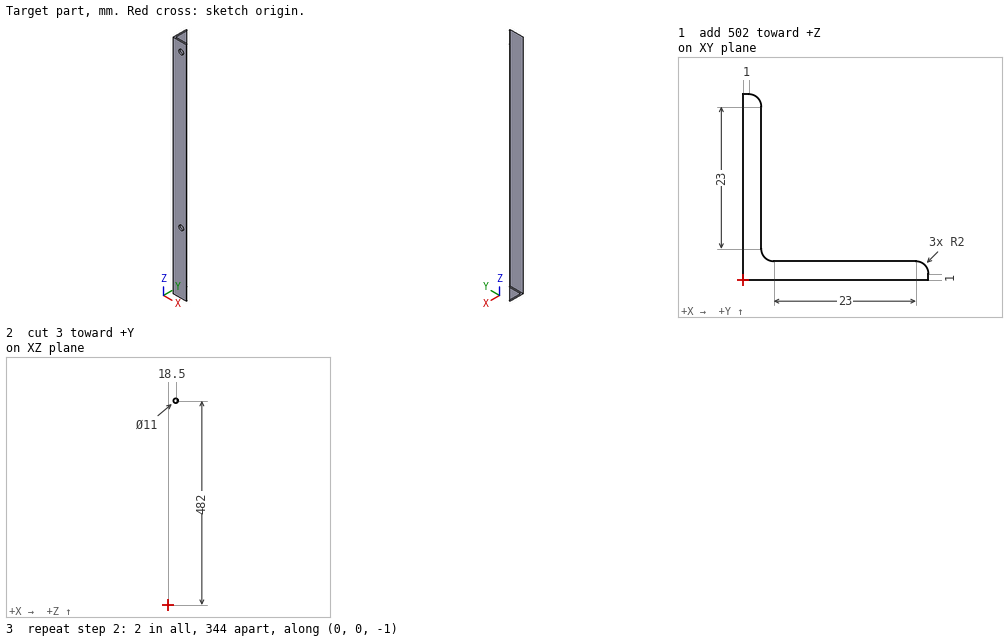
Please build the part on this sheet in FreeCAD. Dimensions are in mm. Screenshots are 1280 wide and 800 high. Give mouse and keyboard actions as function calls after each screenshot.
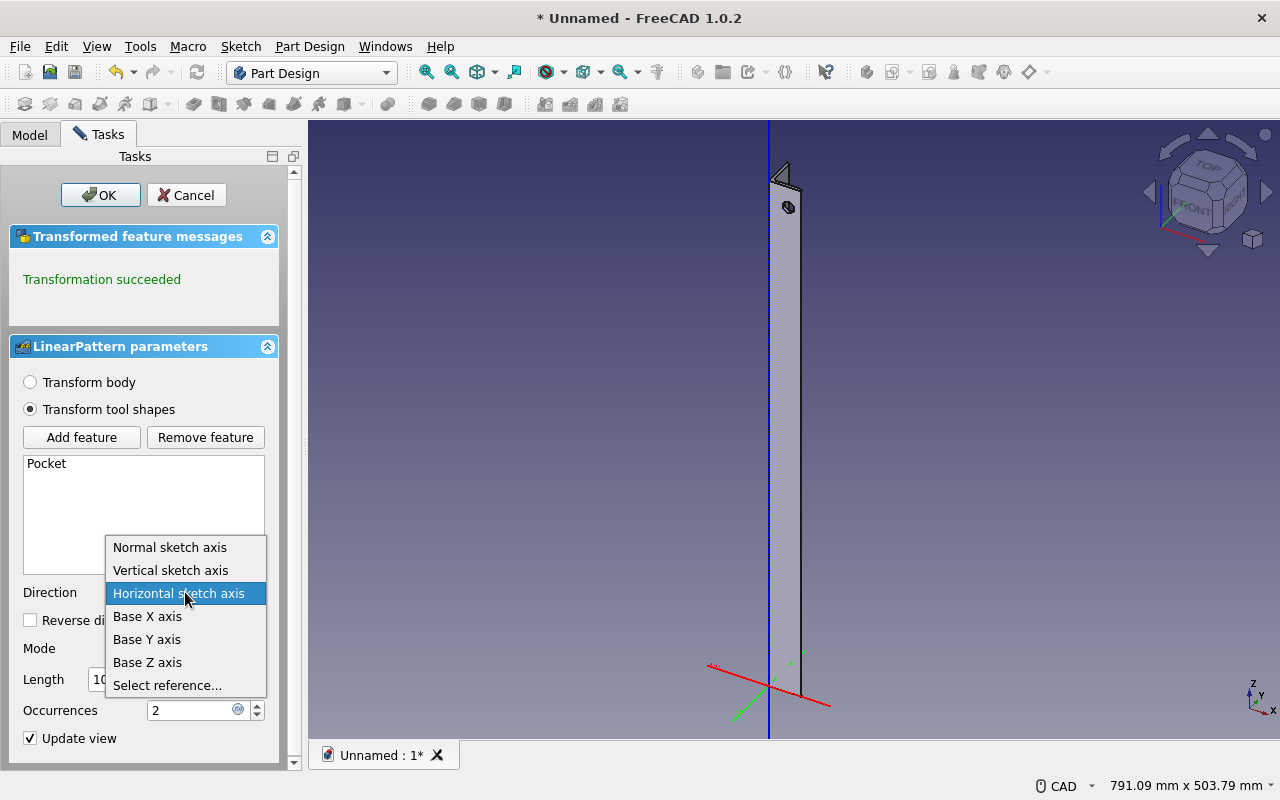
click(184, 662)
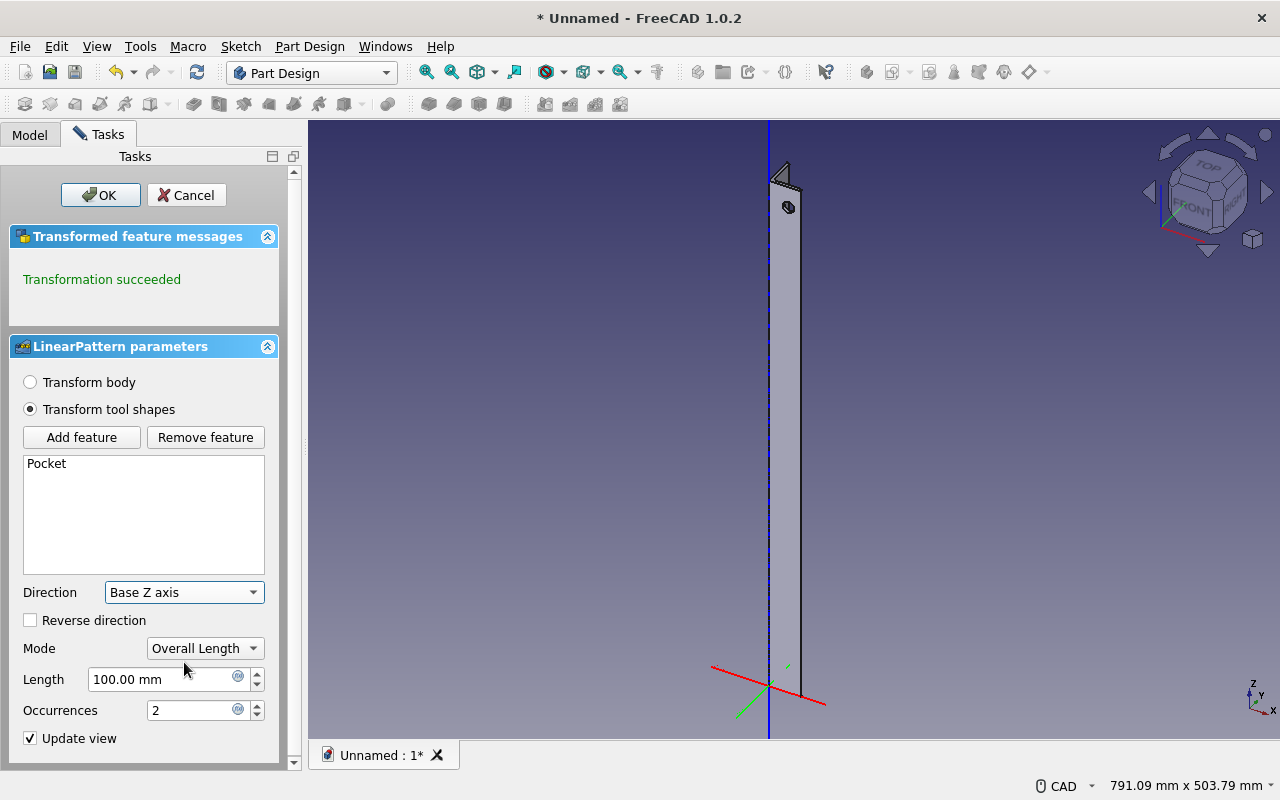
click(206, 648)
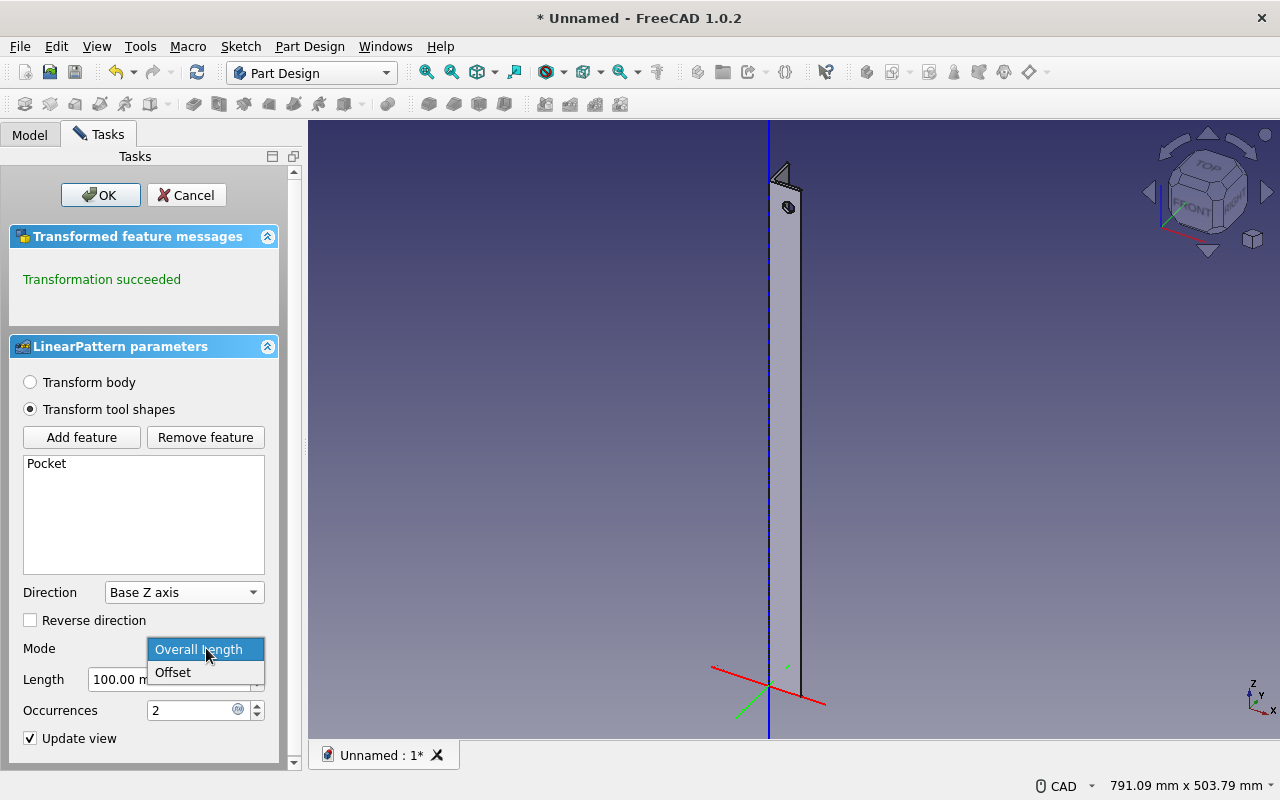
click(204, 672)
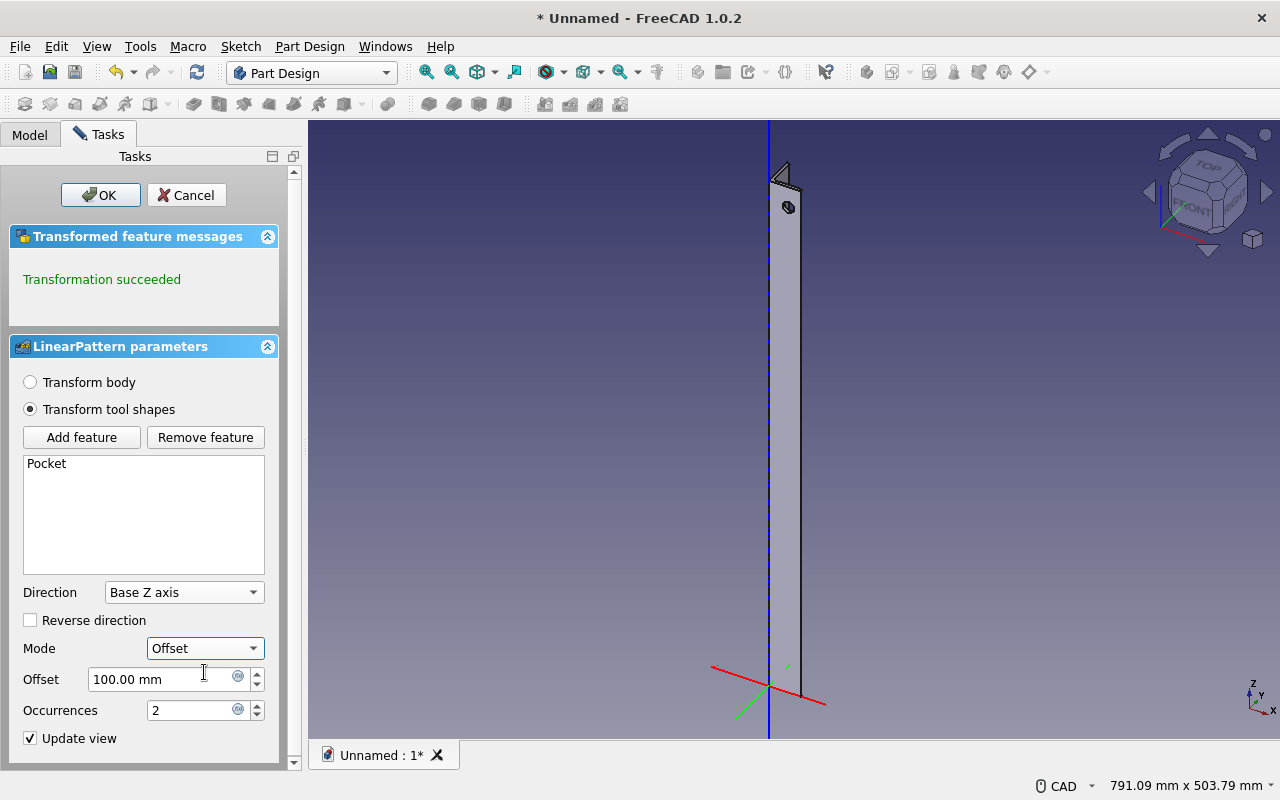
triple_click(170, 680)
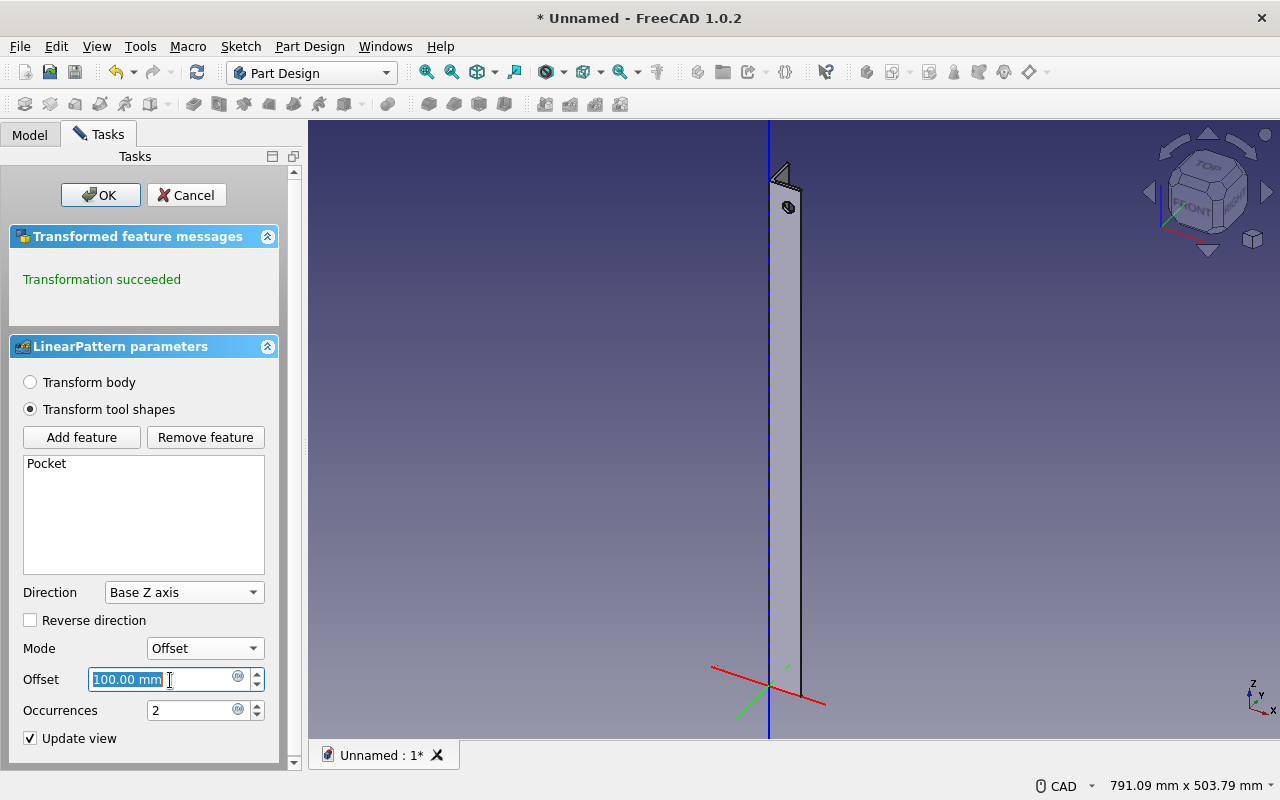
text(344)
key(Tab)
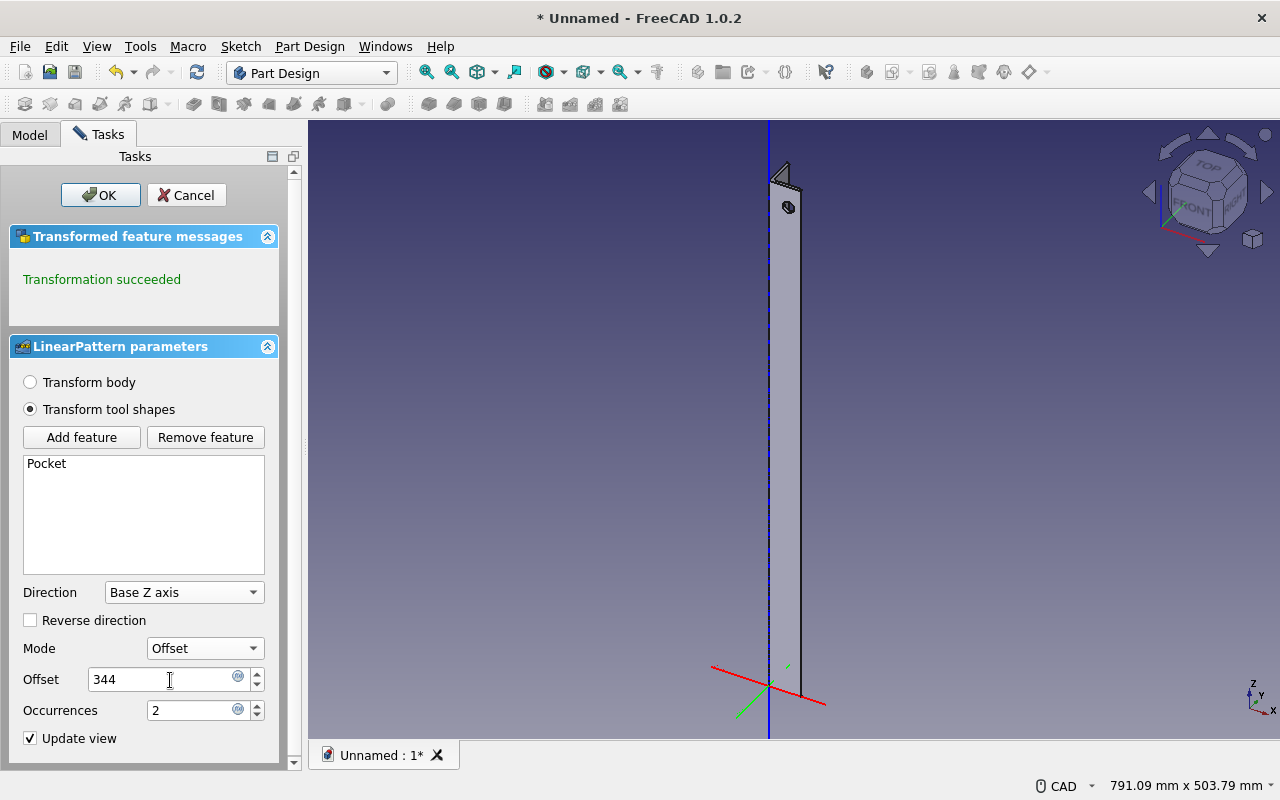
triple_click(199, 710)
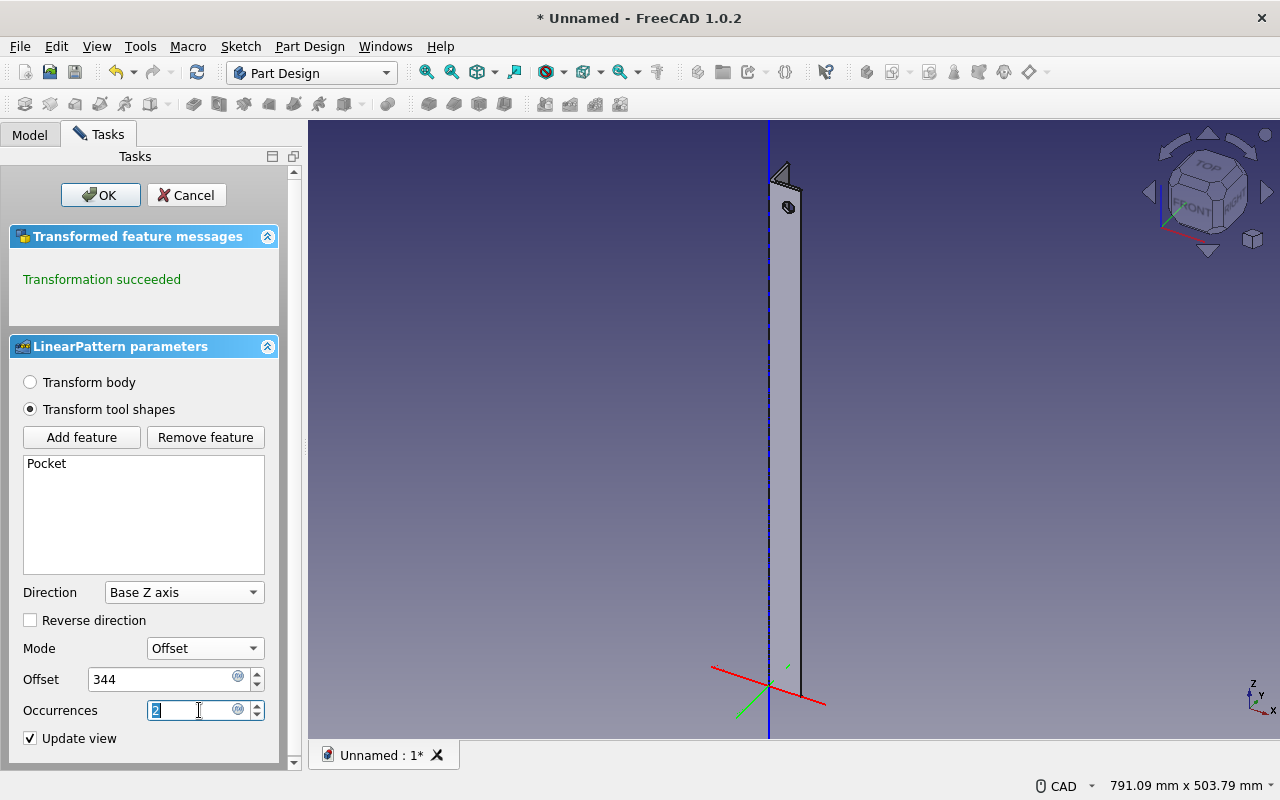
text(2)
key(Tab)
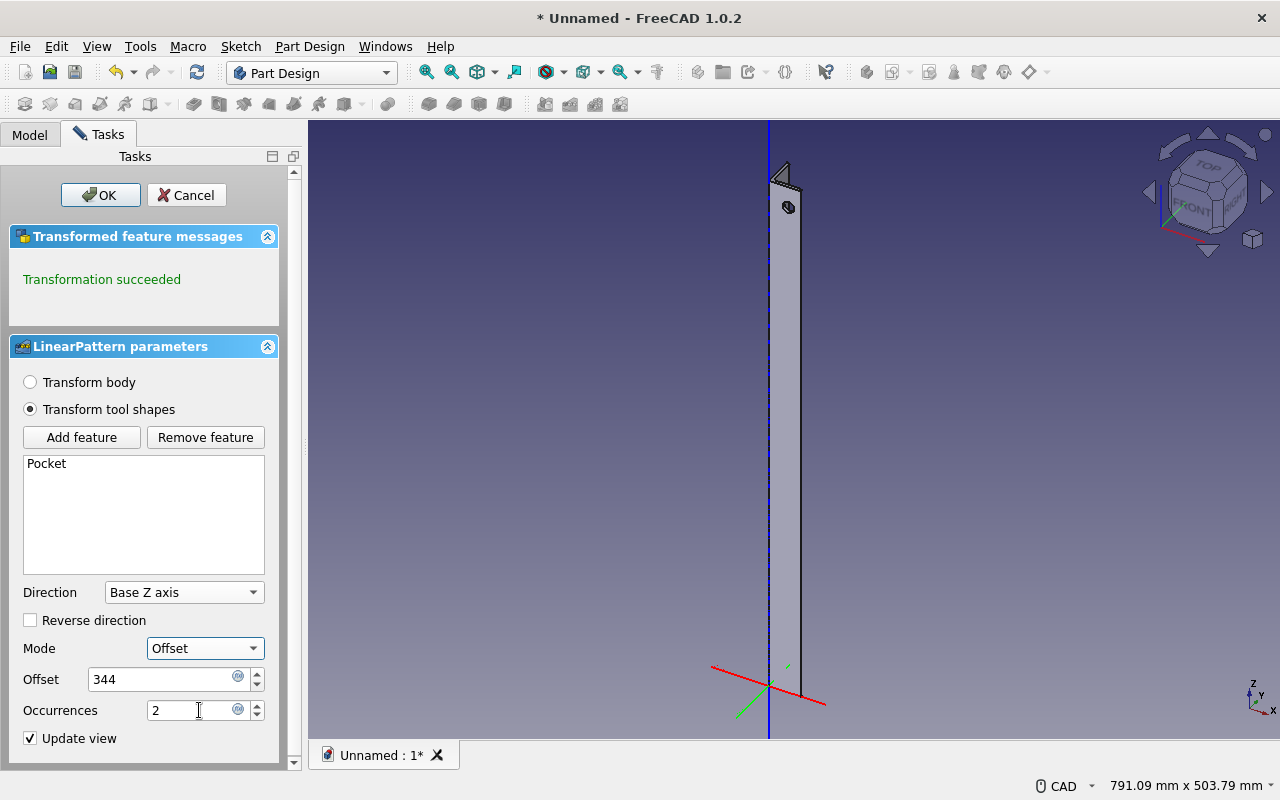
click(31, 620)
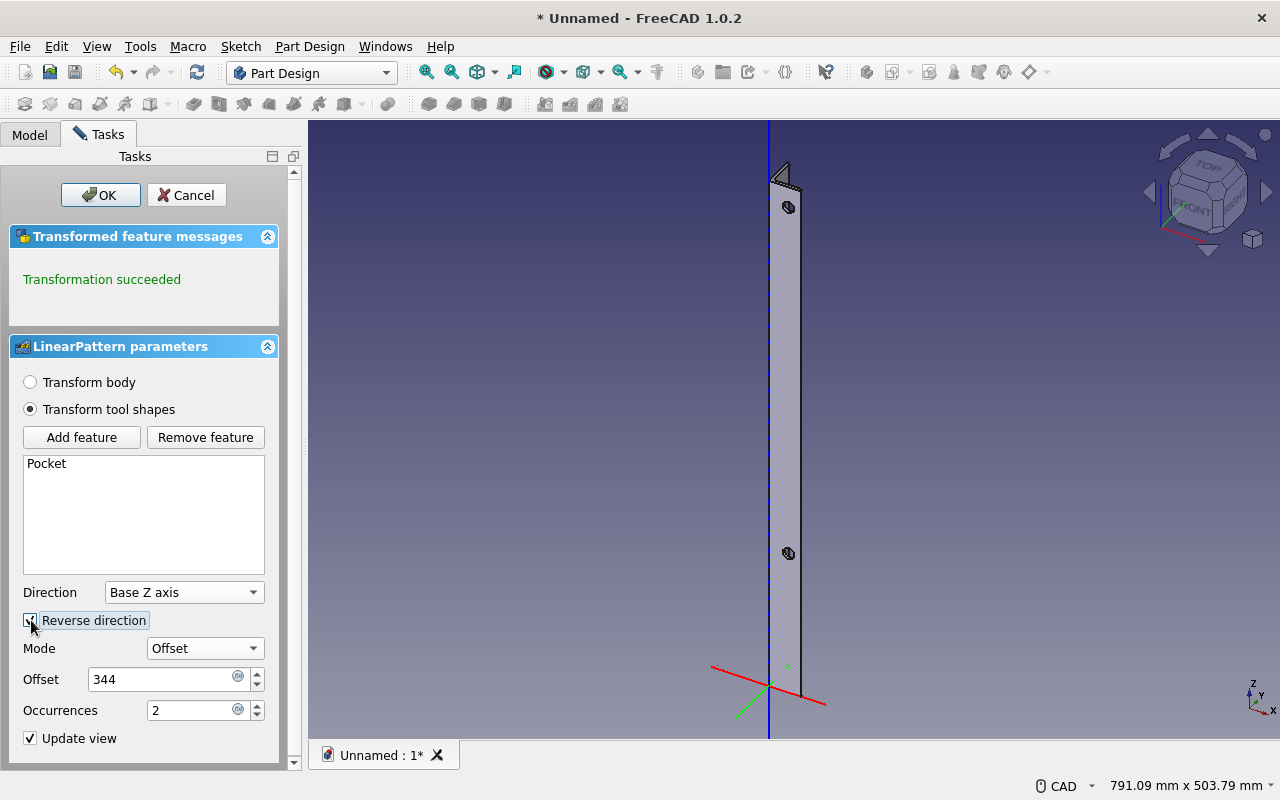
click(101, 195)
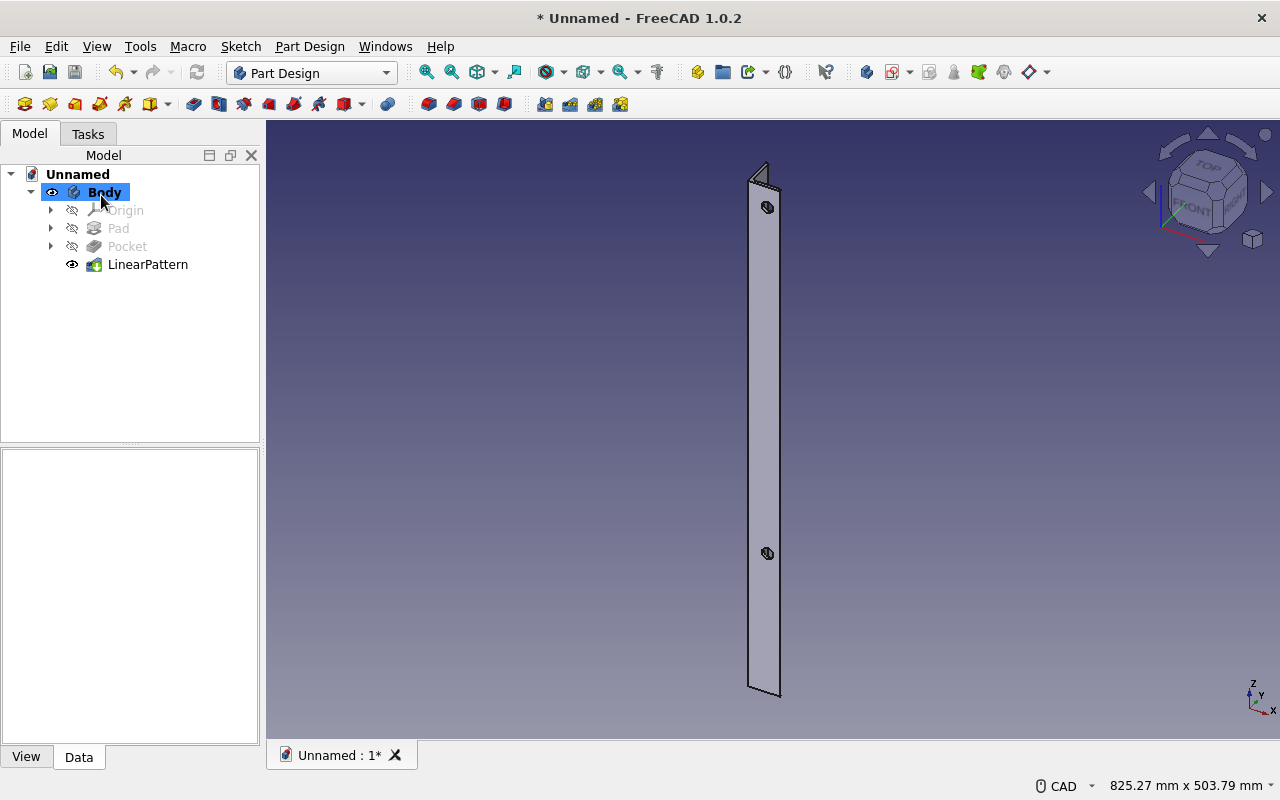
key(0)